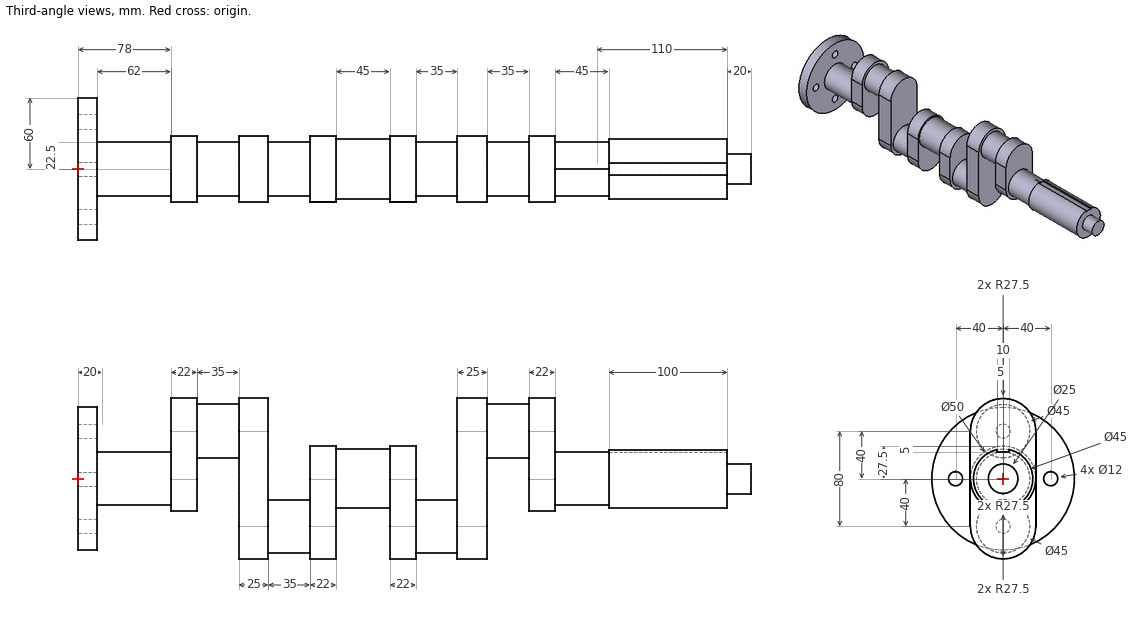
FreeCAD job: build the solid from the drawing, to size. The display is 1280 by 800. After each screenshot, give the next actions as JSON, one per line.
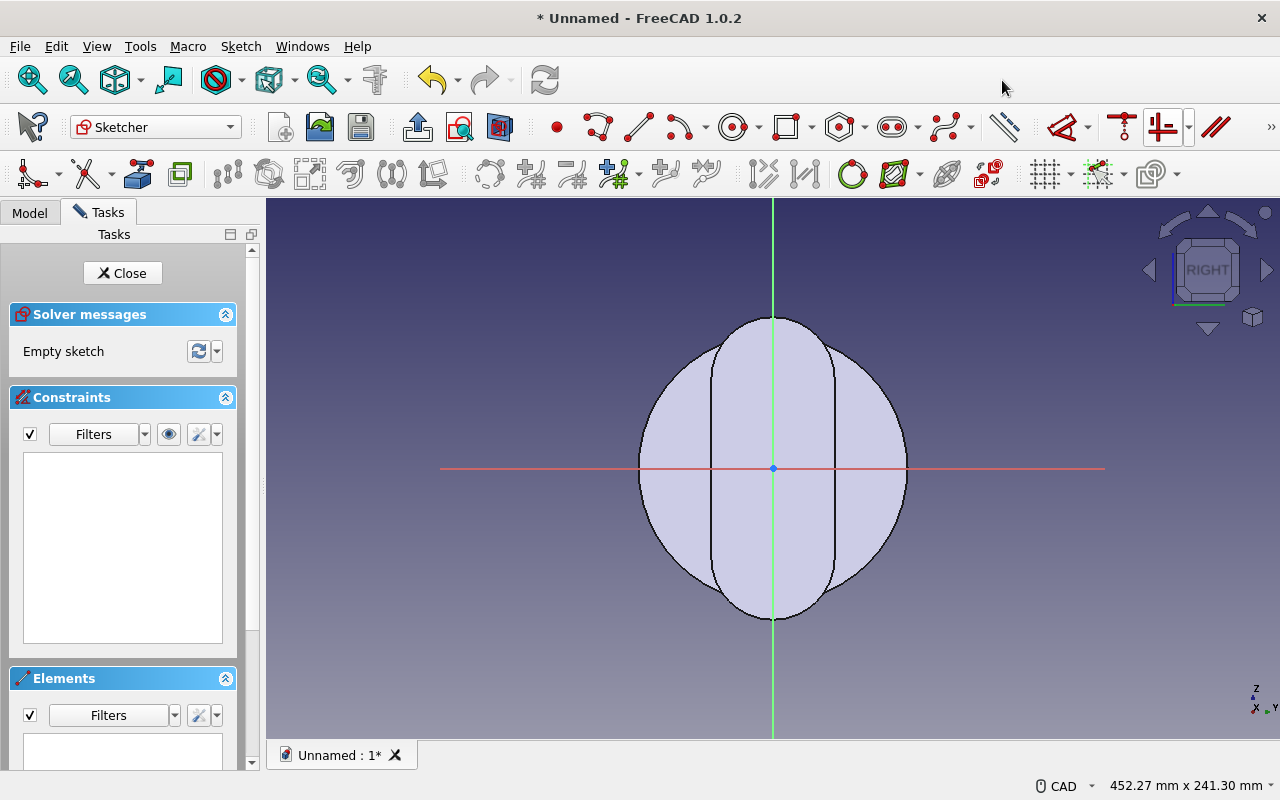
{"action": "scroll", "coordinate": [829, 596], "scroll_direction": "up", "scroll_amount": 4}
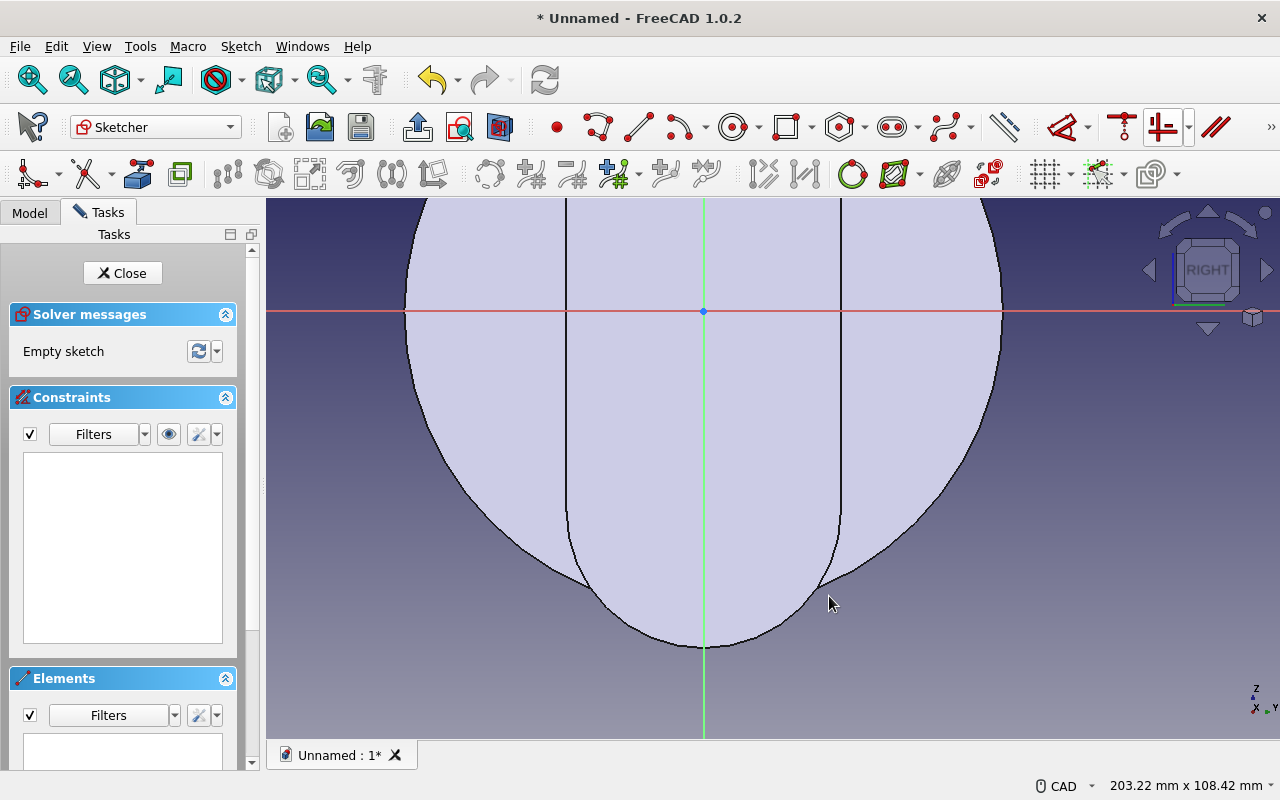
{"action": "left_click", "coordinate": [732, 128]}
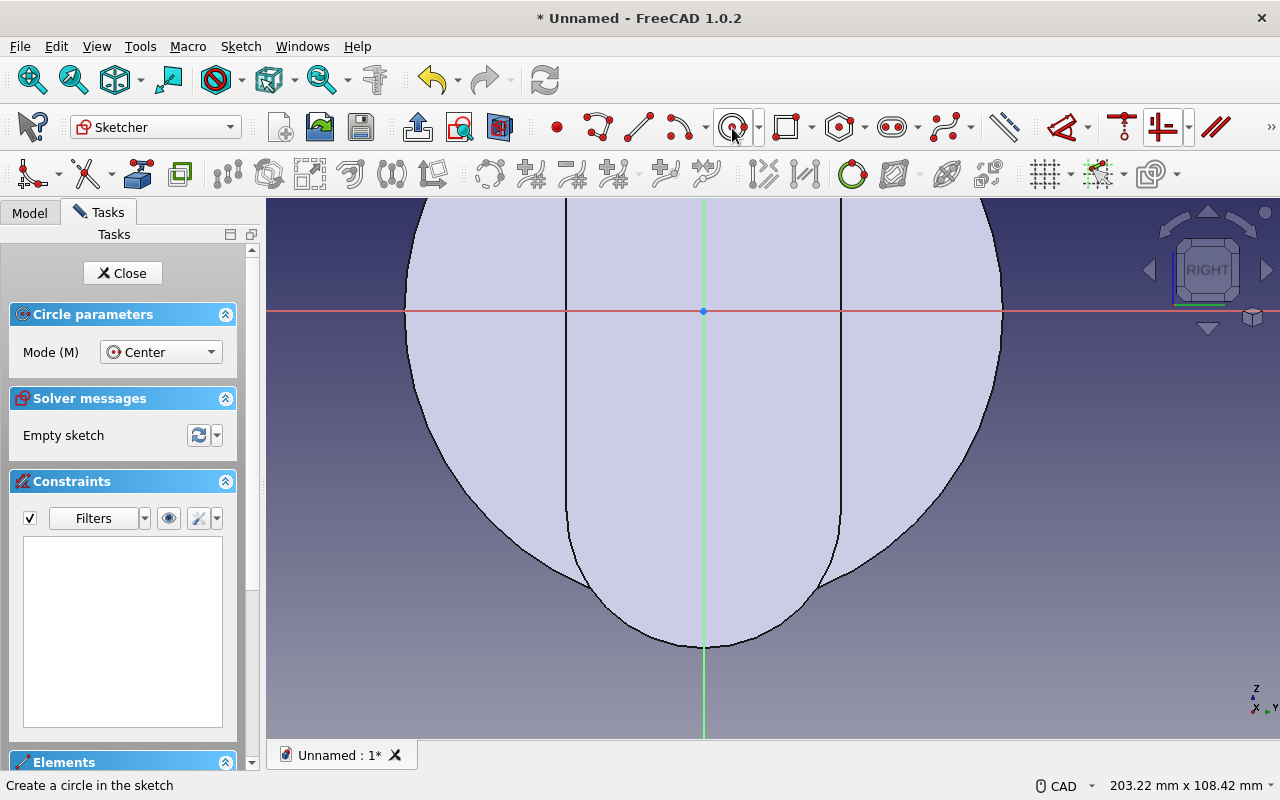
{"action": "left_click", "coordinate": [704, 511]}
{"action": "left_click", "coordinate": [783, 432]}
{"action": "key", "text": "Escape"}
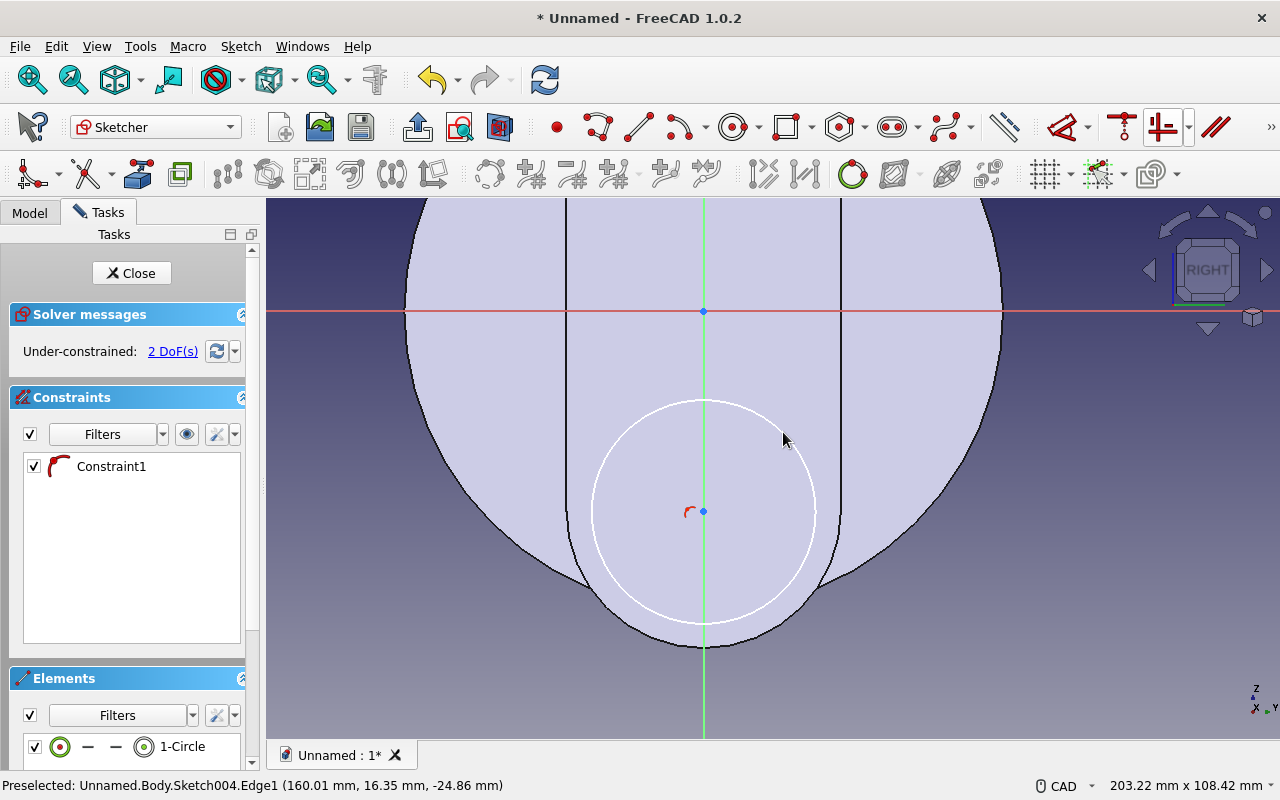
{"action": "left_click", "coordinate": [1062, 128]}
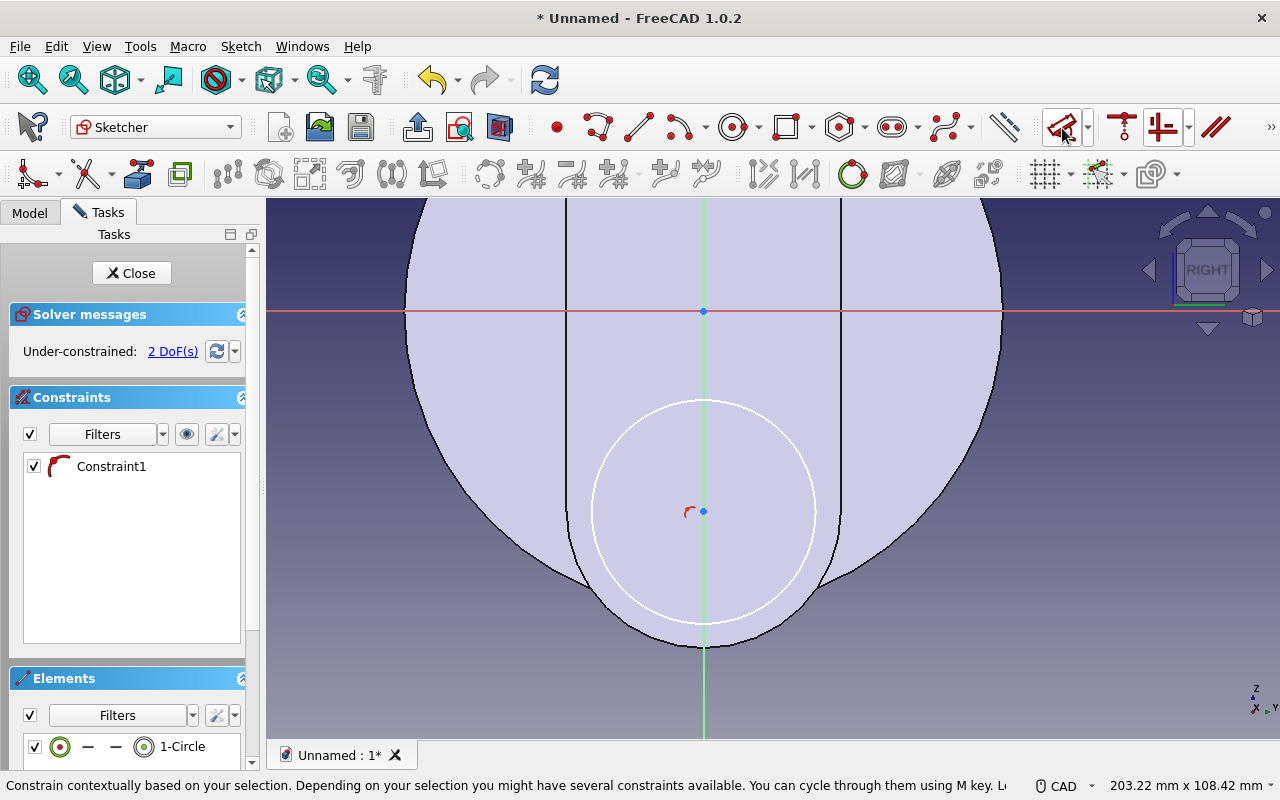
{"action": "left_click", "coordinate": [783, 433]}
{"action": "left_click", "coordinate": [806, 410]}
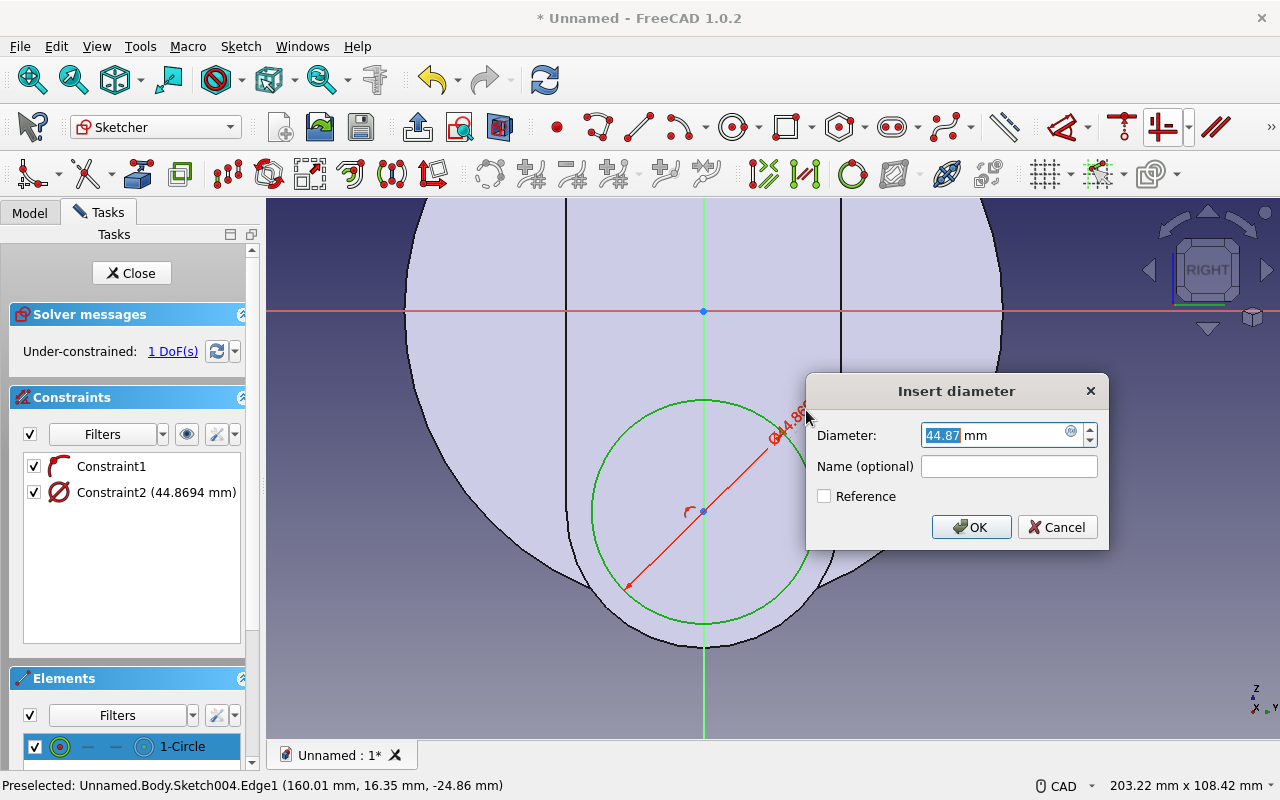
{"action": "type", "text": "45"}
{"action": "key", "text": "Return"}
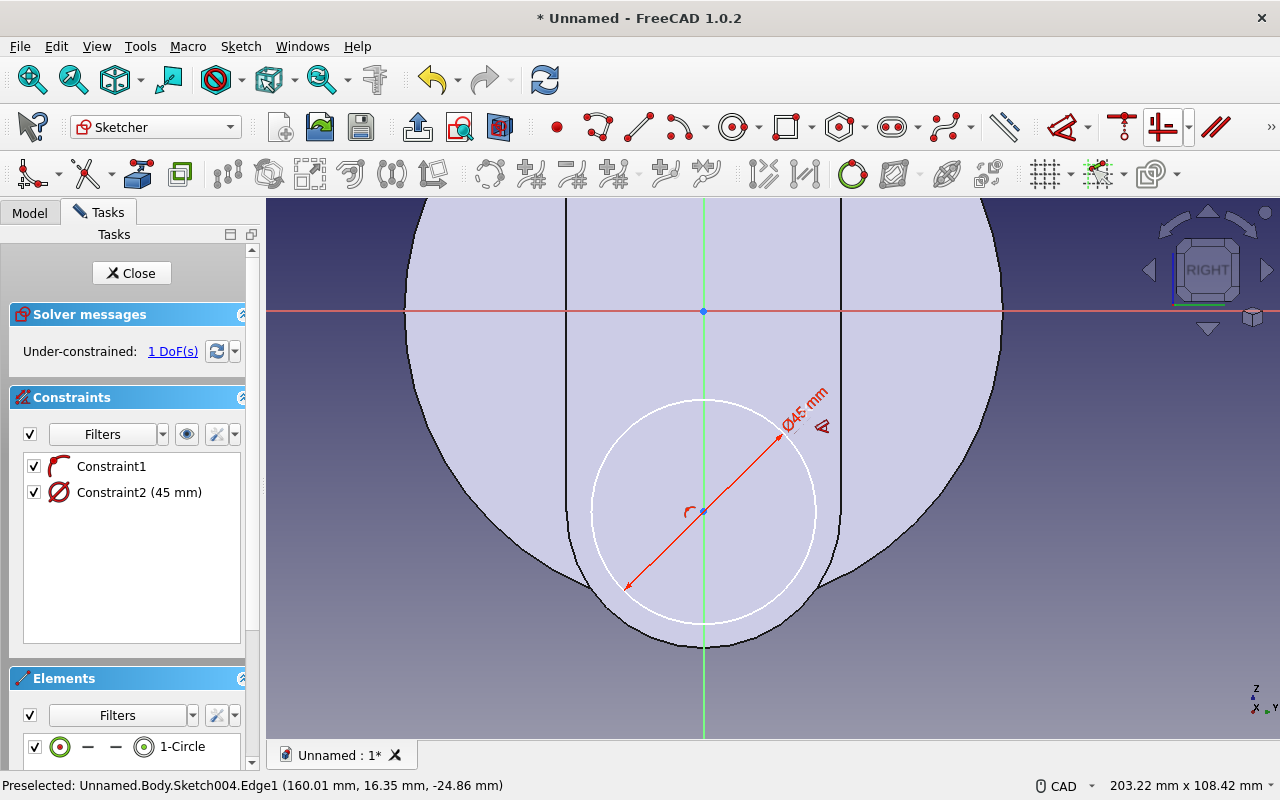
{"action": "left_click", "coordinate": [704, 512]}
{"action": "left_click", "coordinate": [738, 366]}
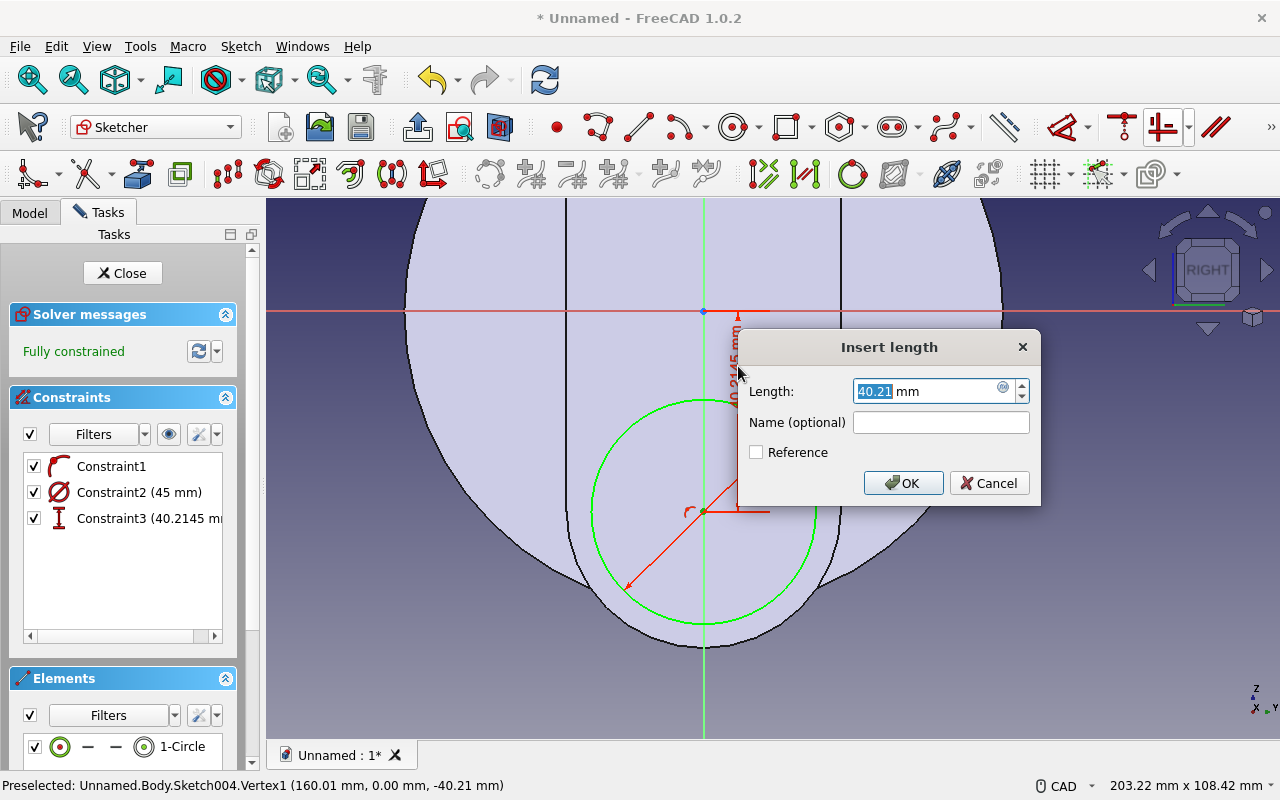
{"action": "type", "text": "40"}
{"action": "key", "text": "Return"}
{"action": "key", "text": "Escape"}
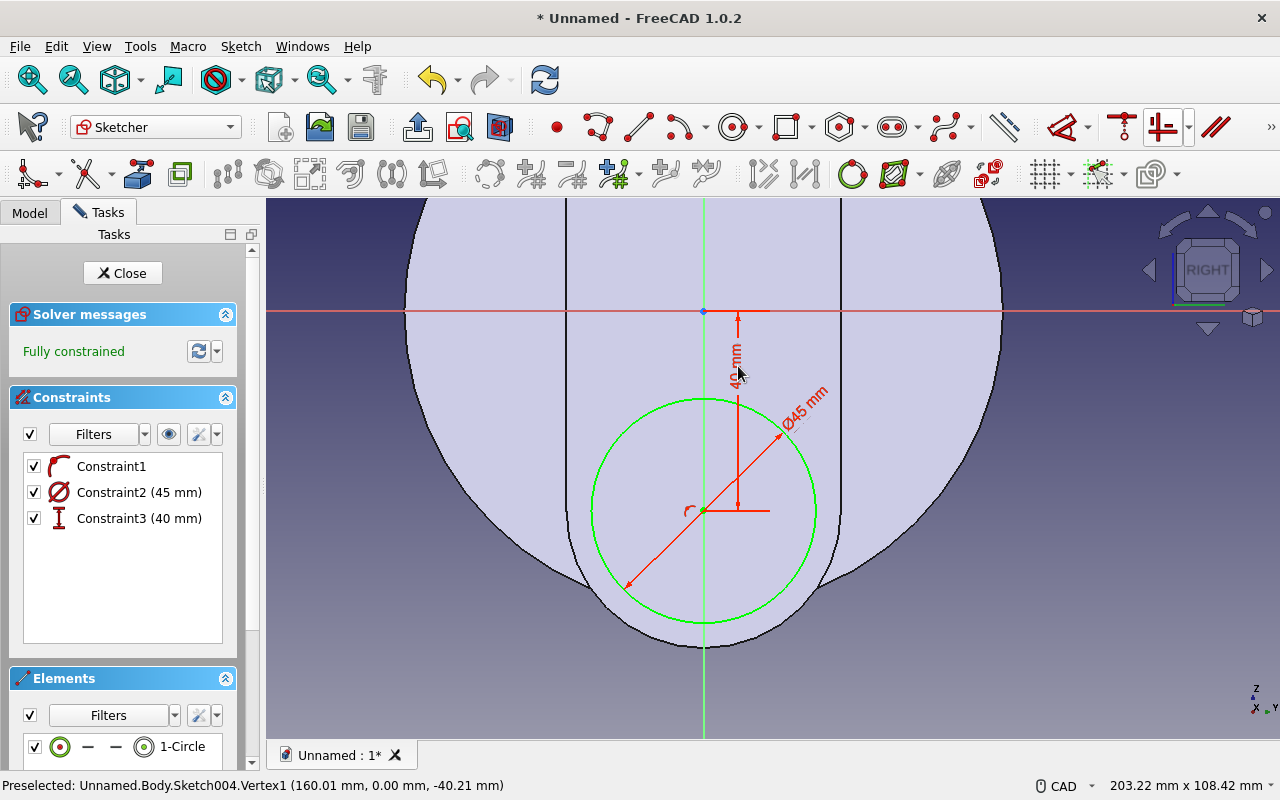
{"action": "left_click", "coordinate": [123, 273]}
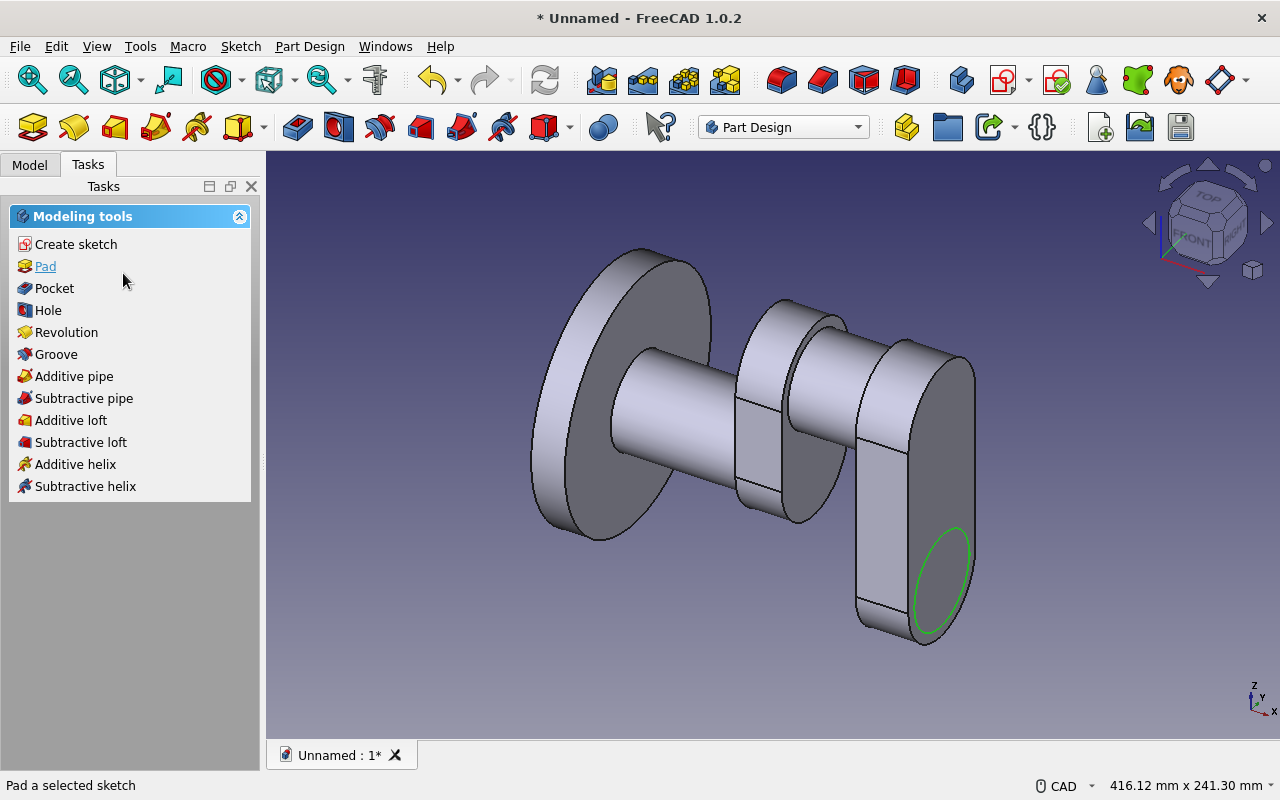
{"action": "left_click", "coordinate": [33, 128]}